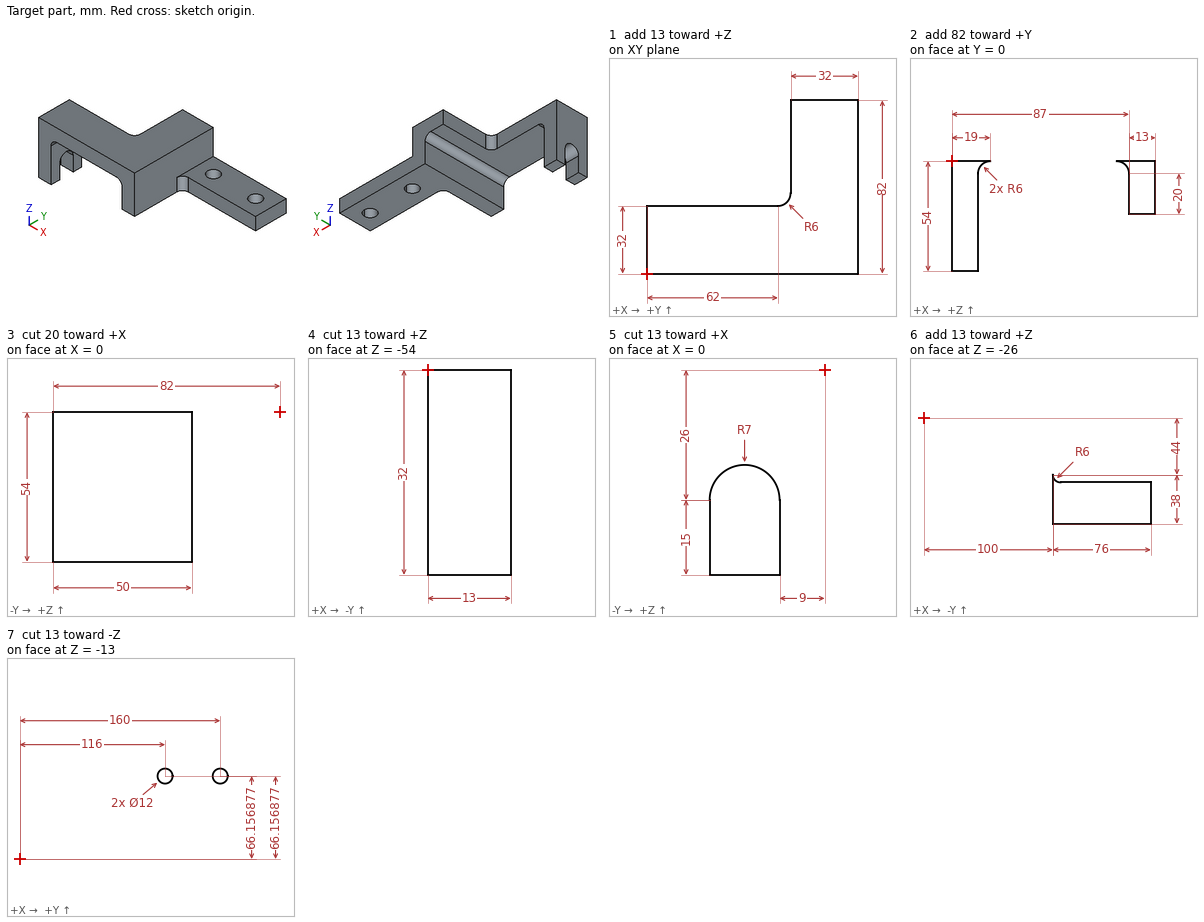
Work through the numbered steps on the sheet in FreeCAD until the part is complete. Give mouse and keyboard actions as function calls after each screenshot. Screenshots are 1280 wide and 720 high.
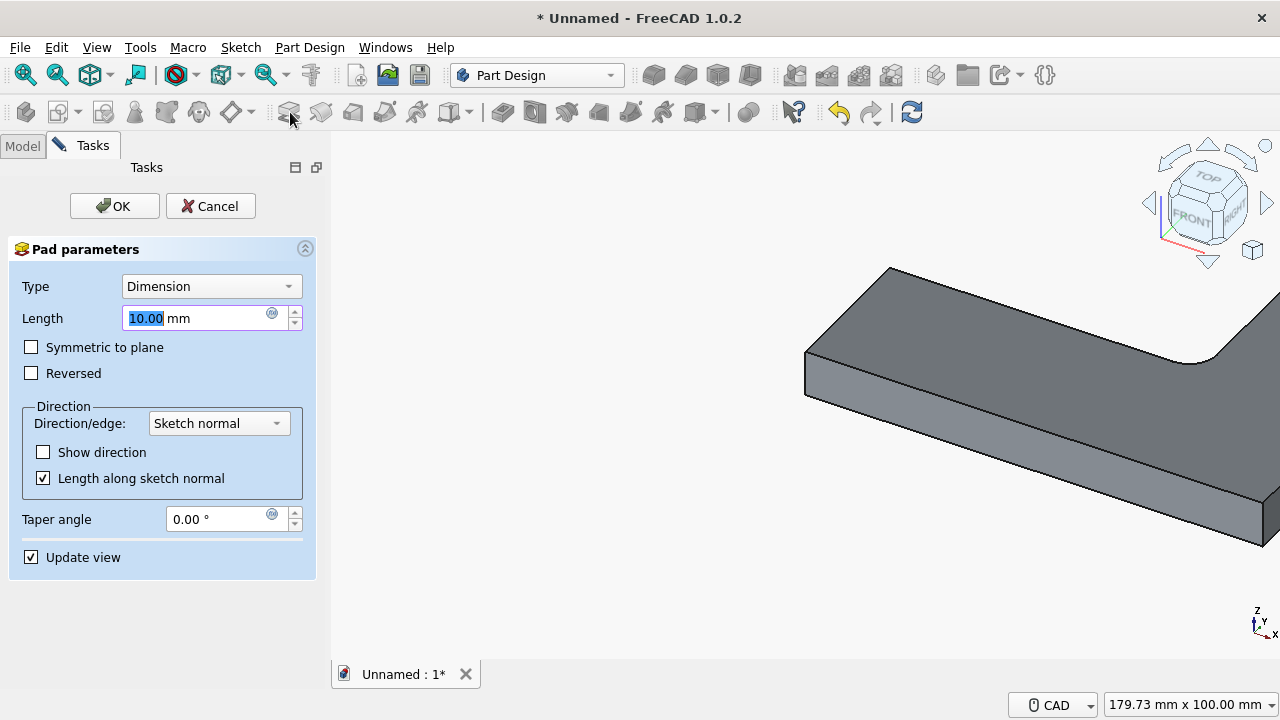
text(13)
key(Tab)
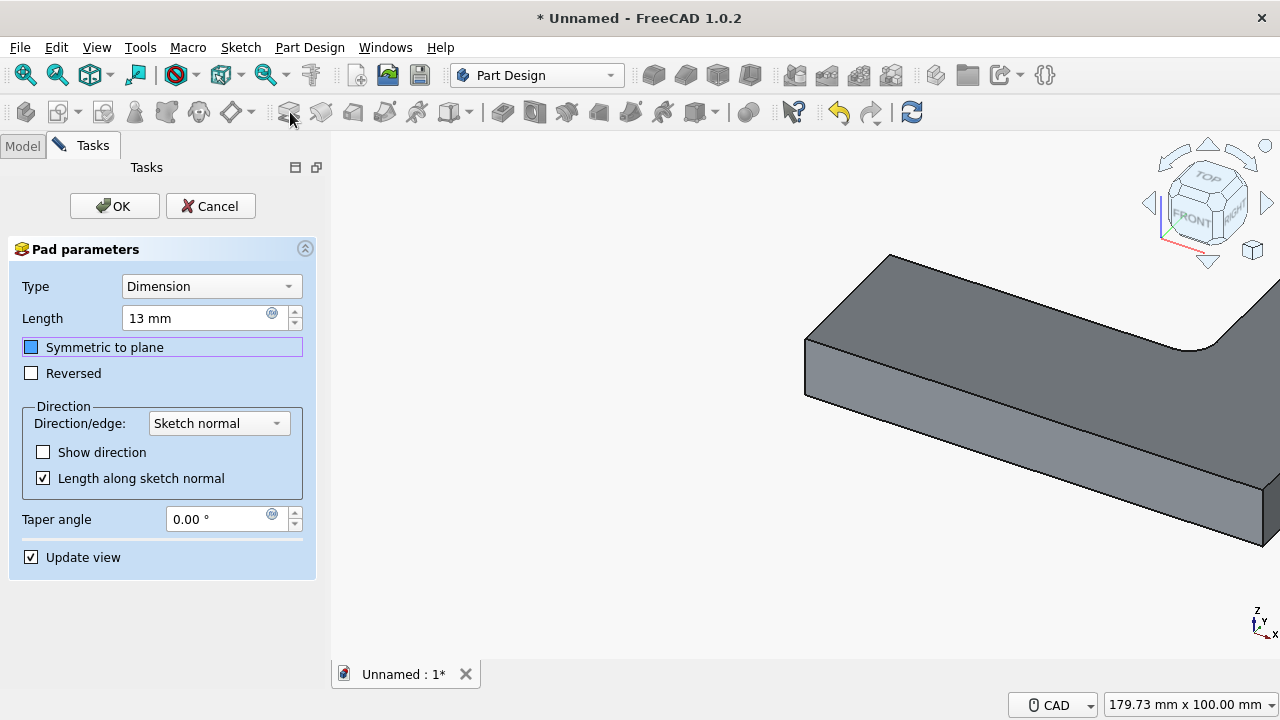
click(115, 206)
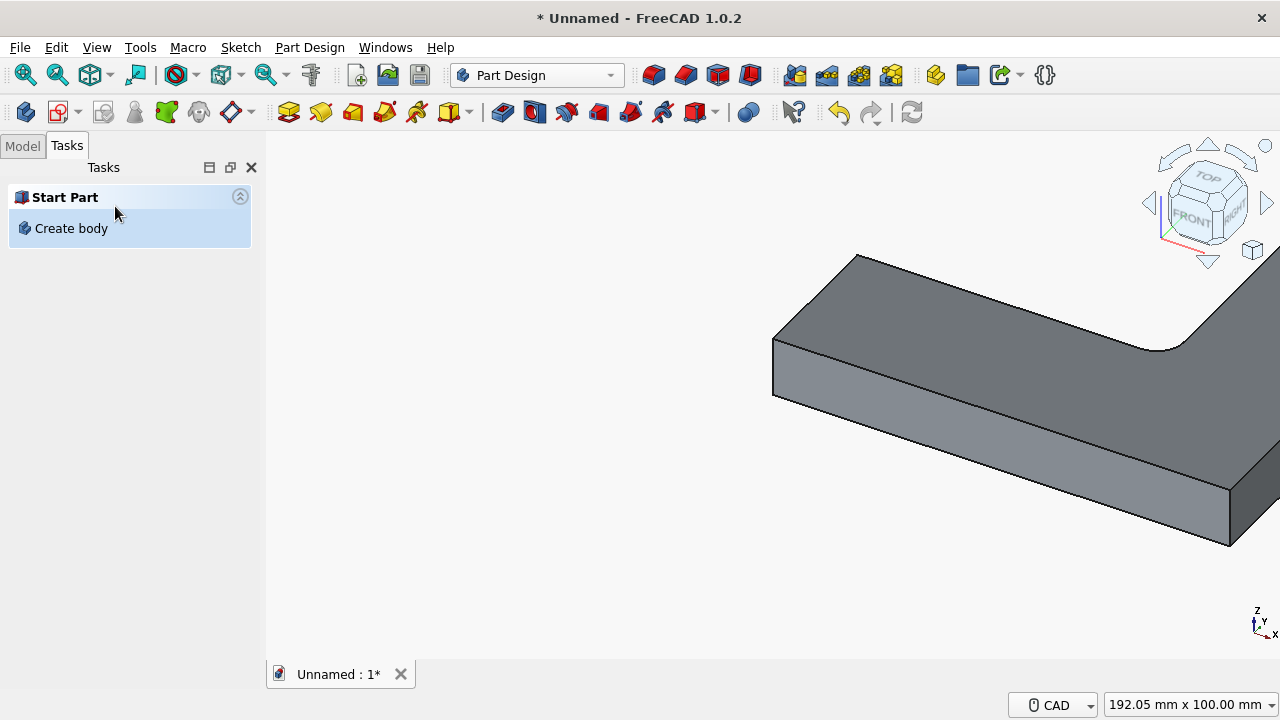
click(26, 76)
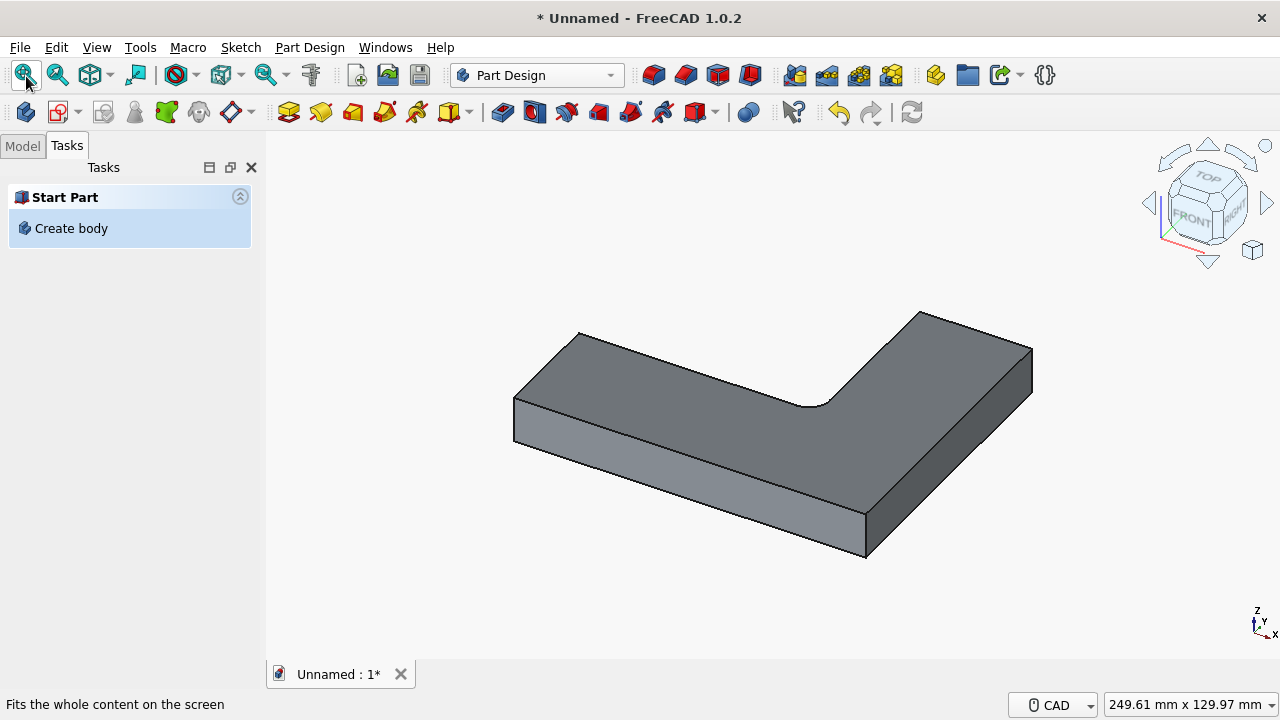
click(840, 527)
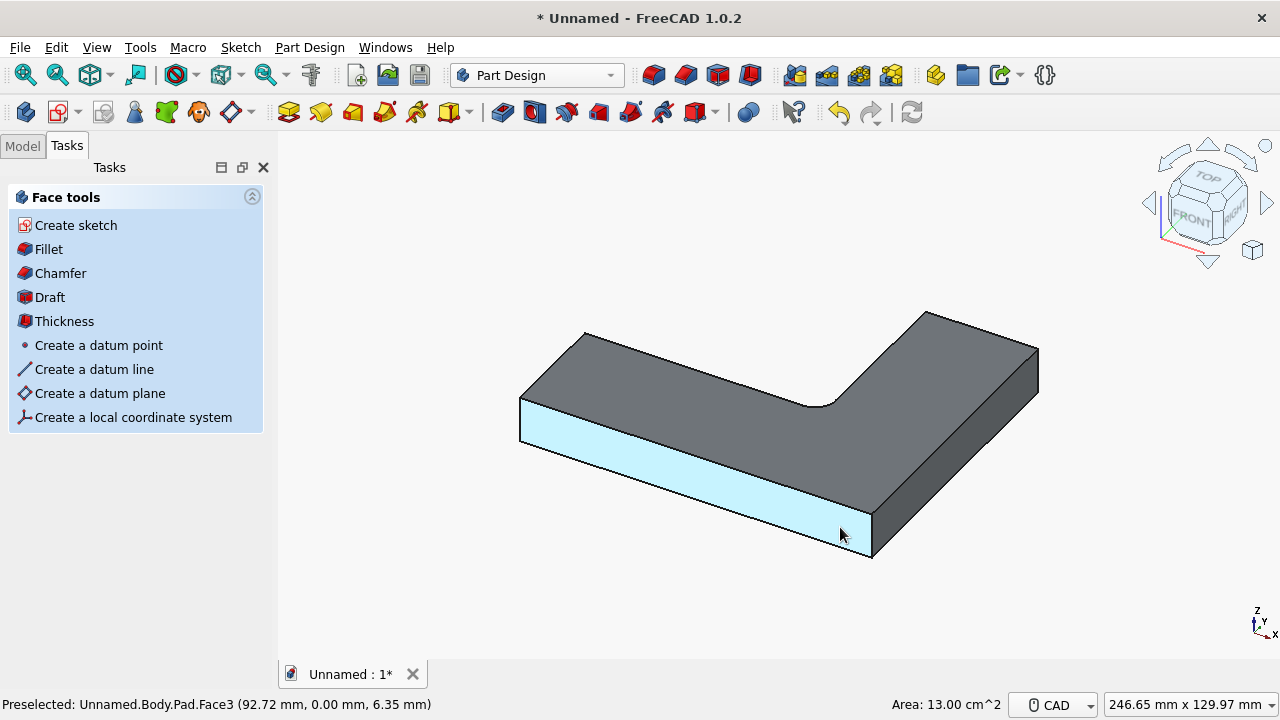
click(58, 112)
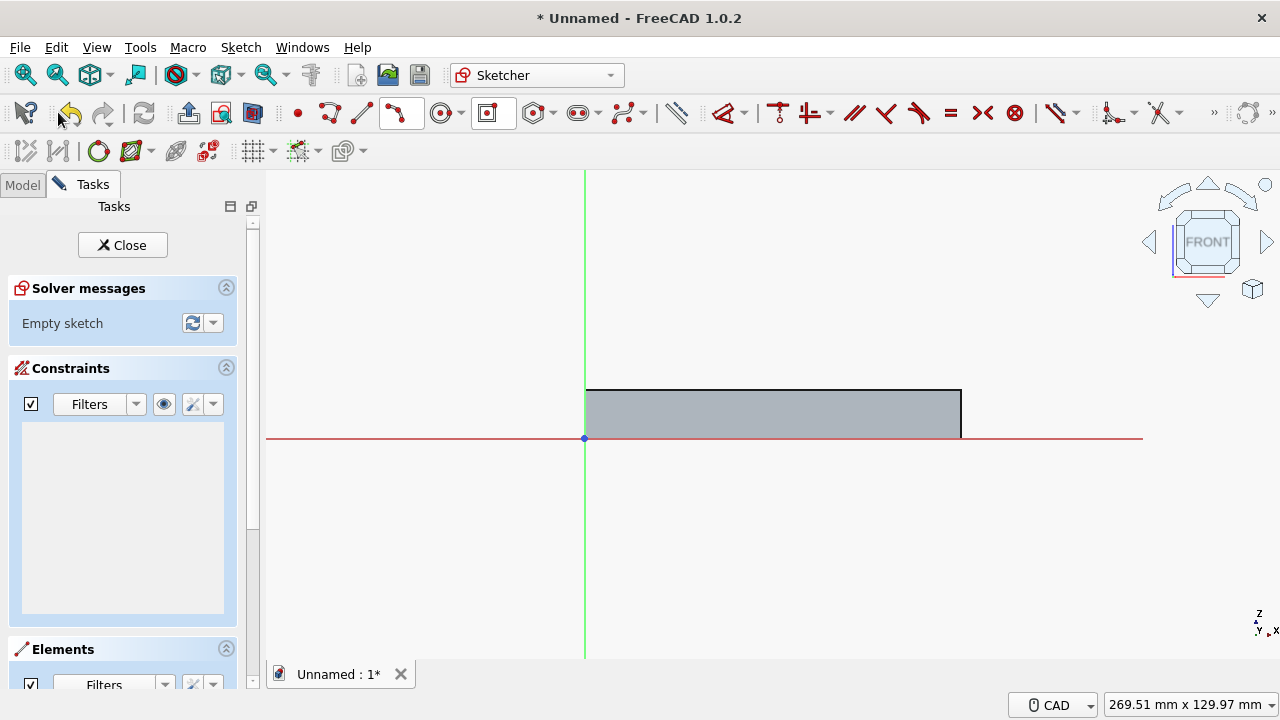
scroll(395, 198, down, 1)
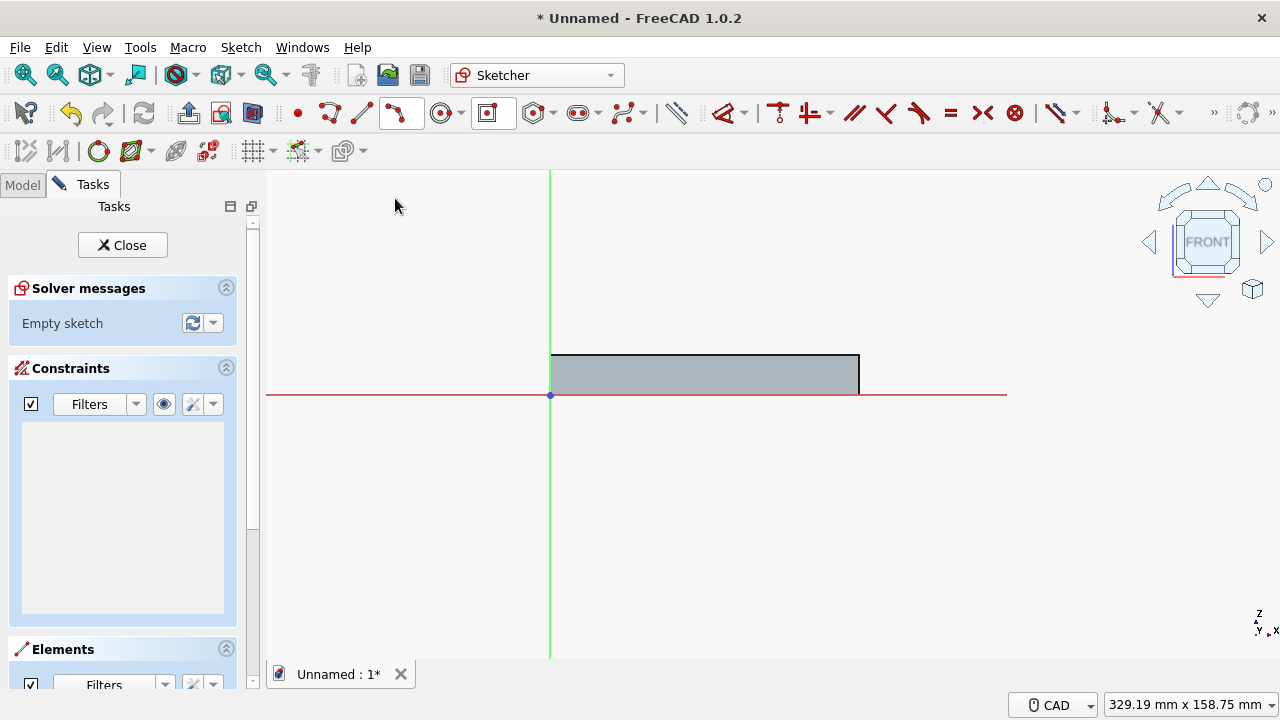
scroll(705, 556, up, 3)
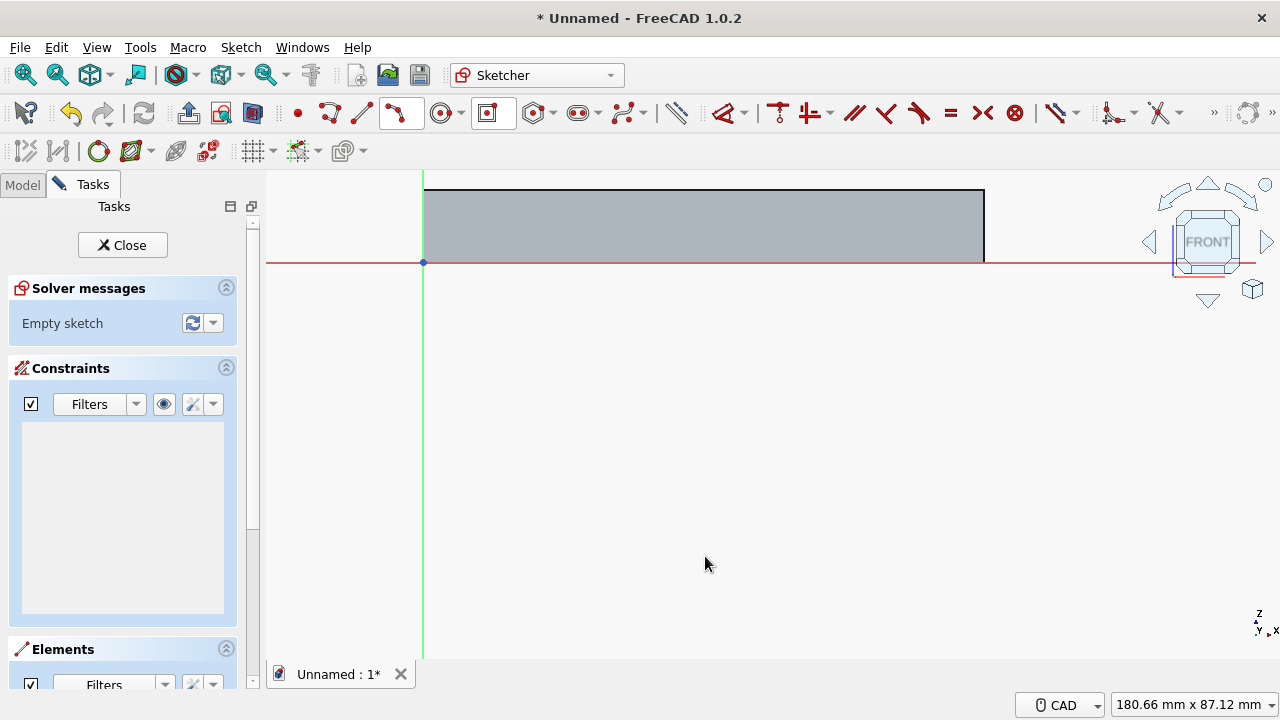
click(330, 114)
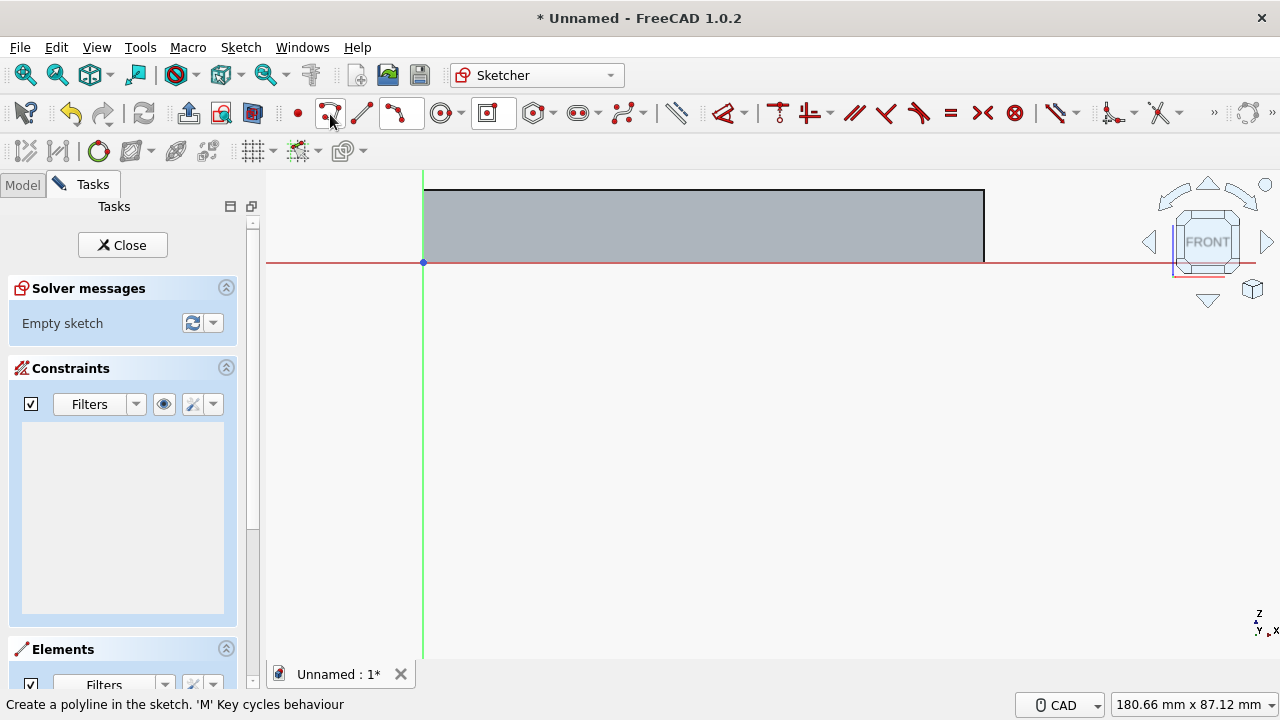
click(530, 263)
click(423, 263)
click(432, 566)
click(496, 566)
click(496, 296)
right_click(496, 296)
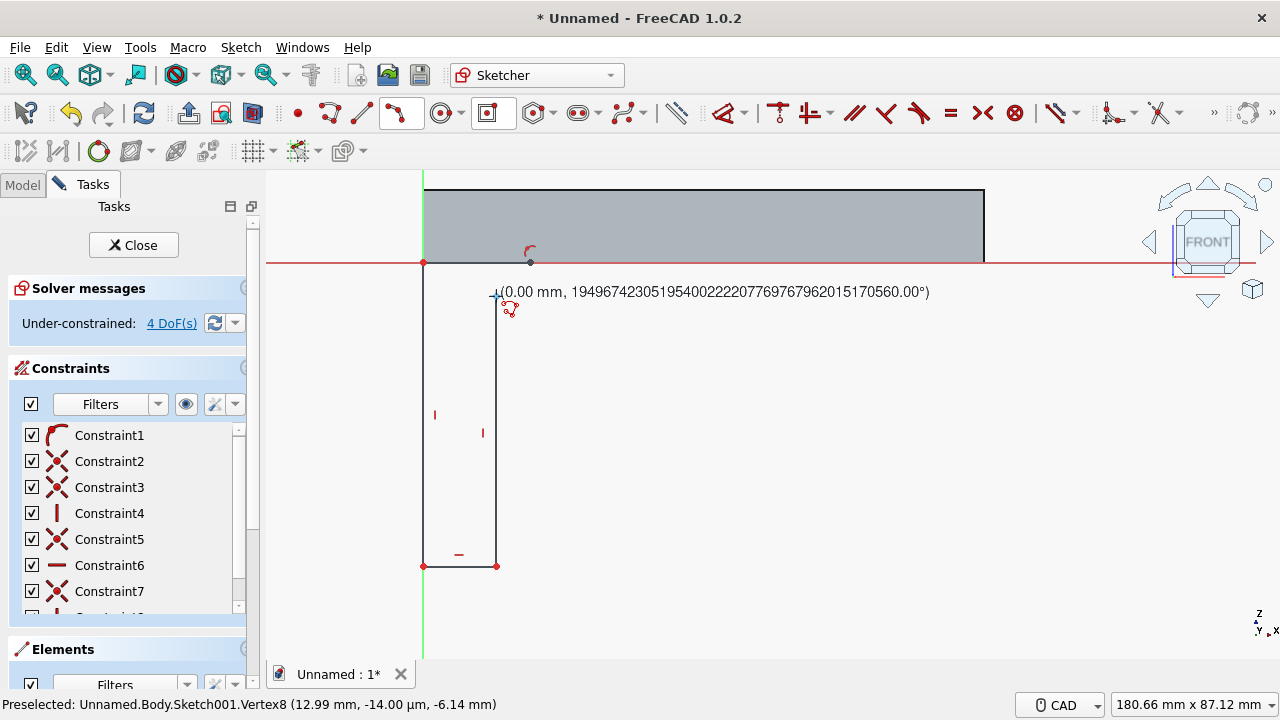
click(396, 114)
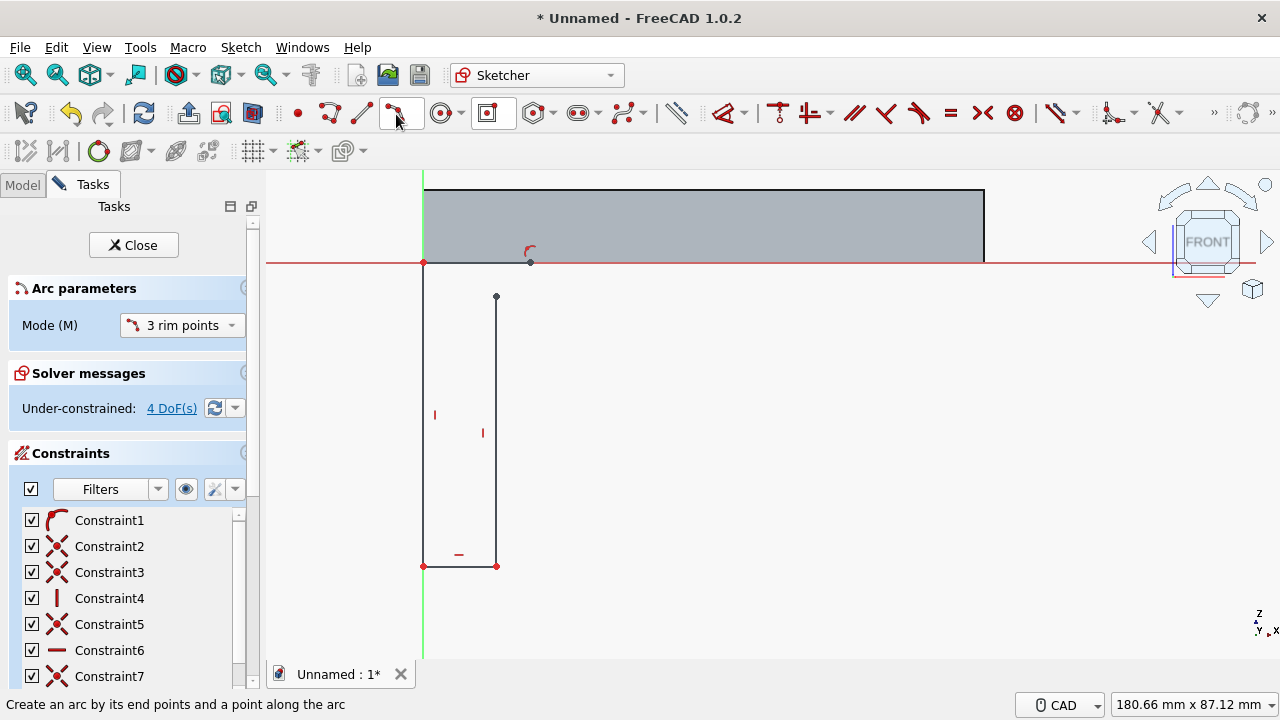
click(496, 297)
click(530, 263)